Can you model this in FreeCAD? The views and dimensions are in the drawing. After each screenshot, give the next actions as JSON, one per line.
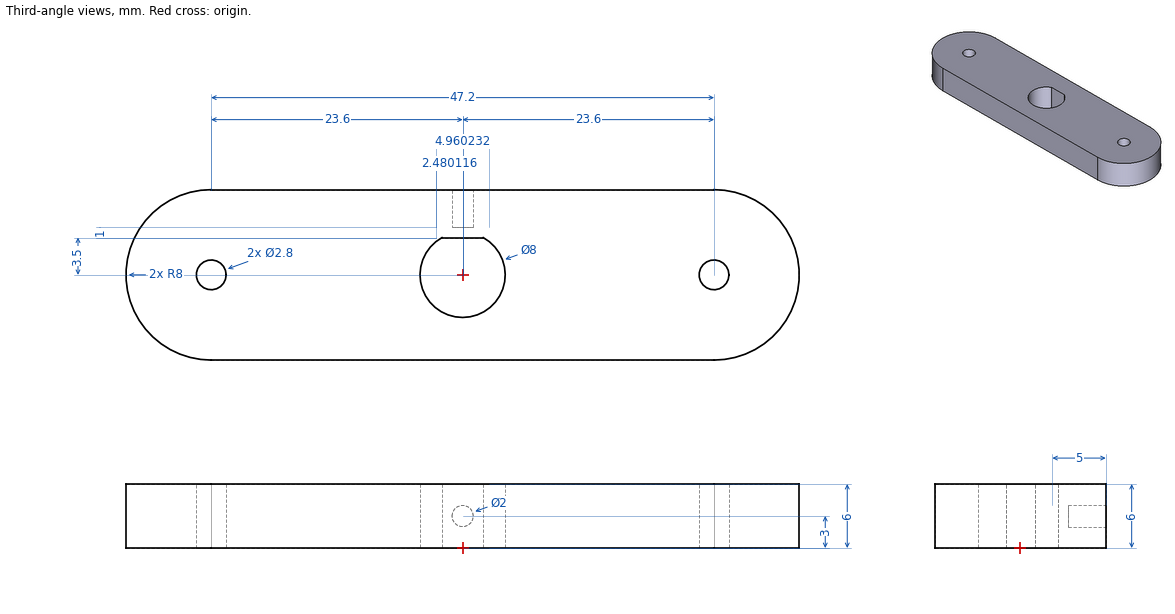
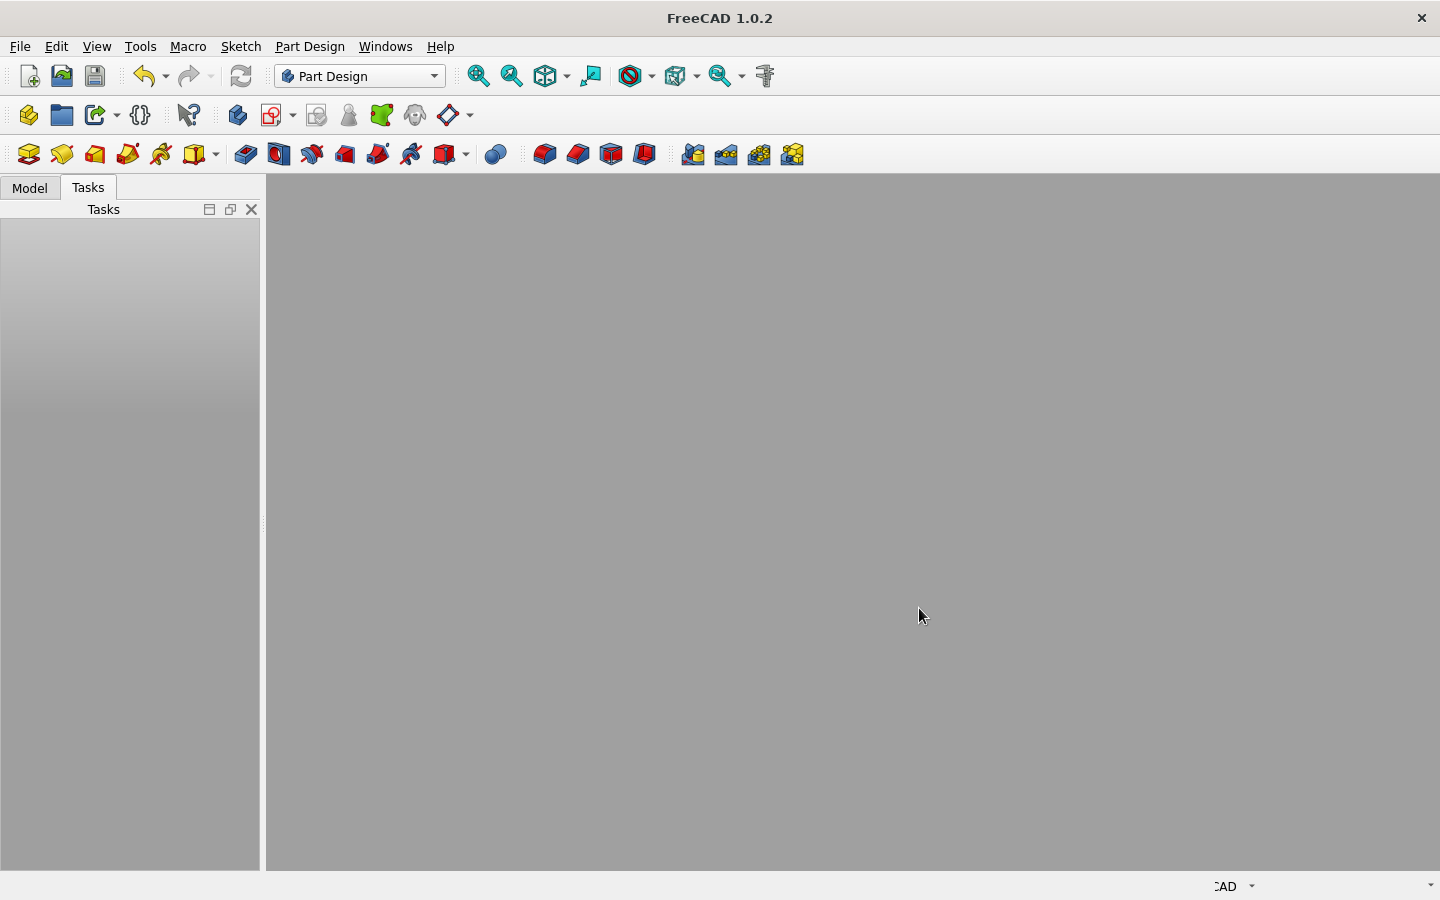
{"action": "left_click", "coordinate": [29, 76]}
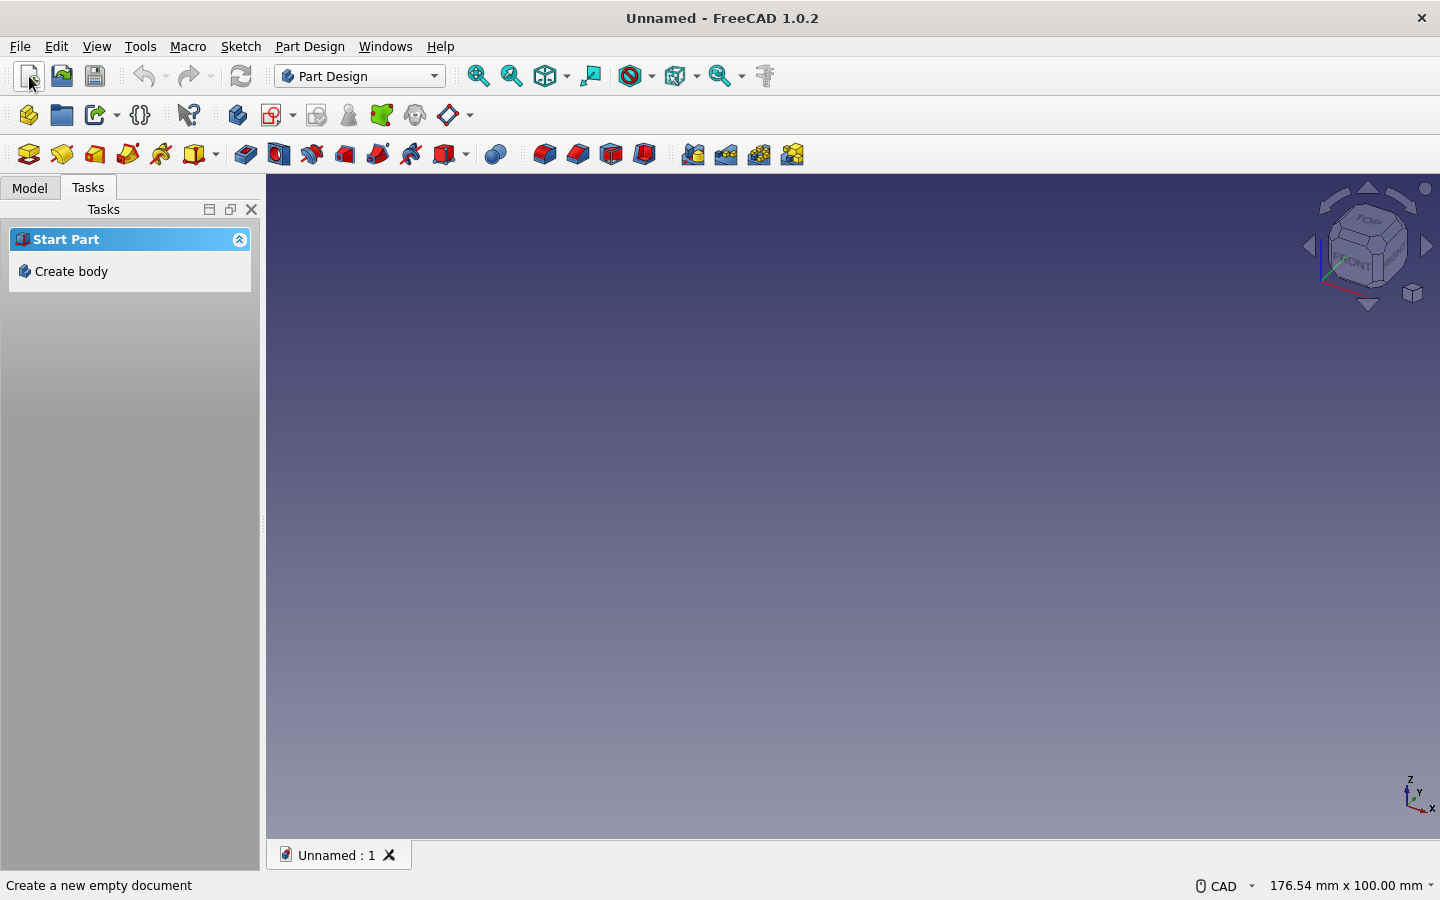
{"action": "left_click", "coordinate": [270, 116]}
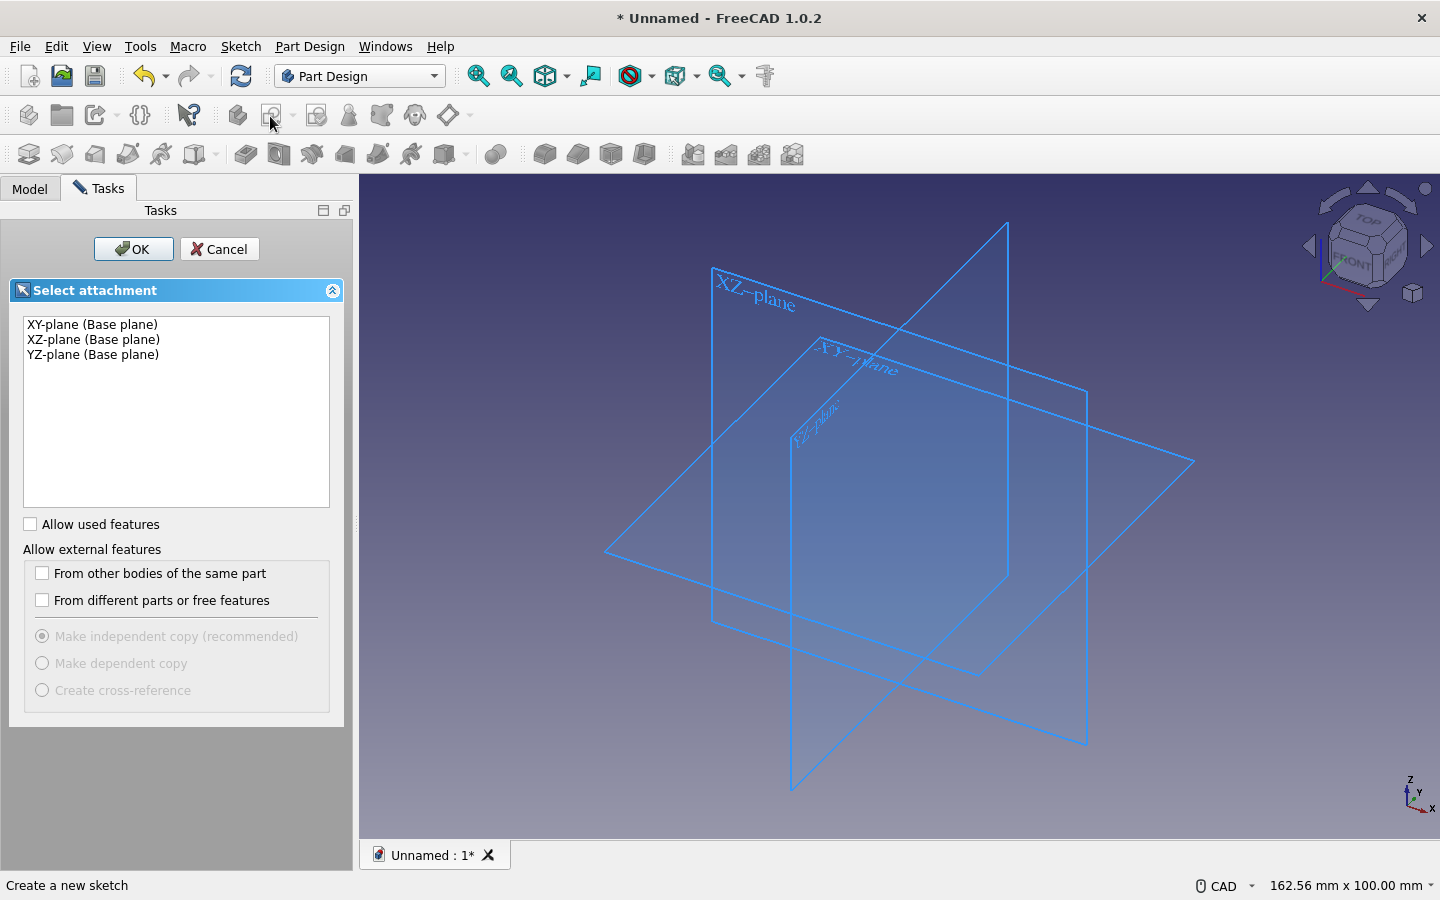
{"action": "left_click", "coordinate": [84, 324]}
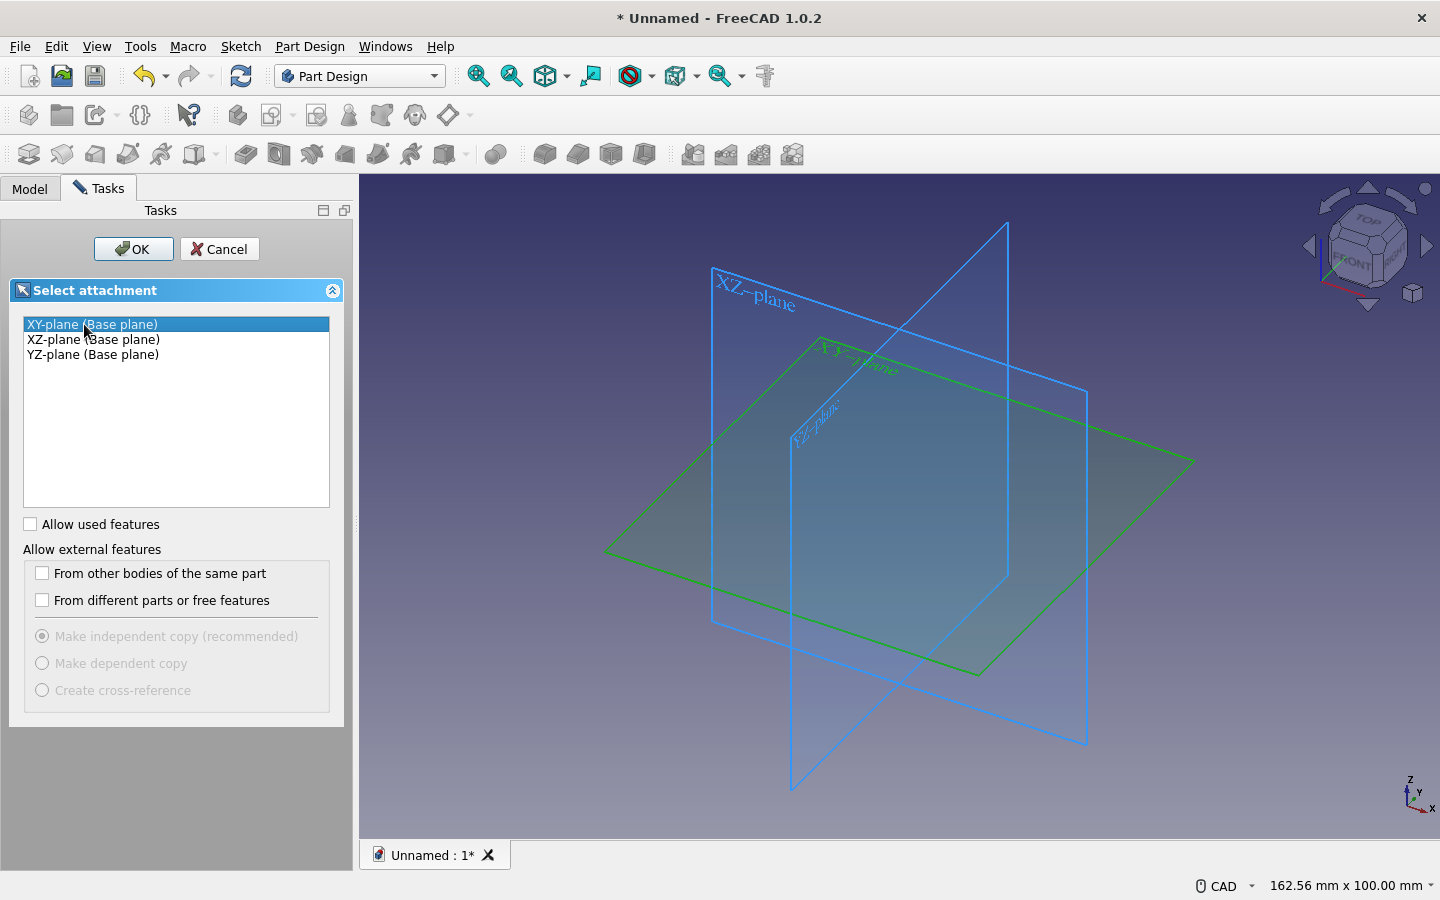
{"action": "left_click", "coordinate": [134, 249]}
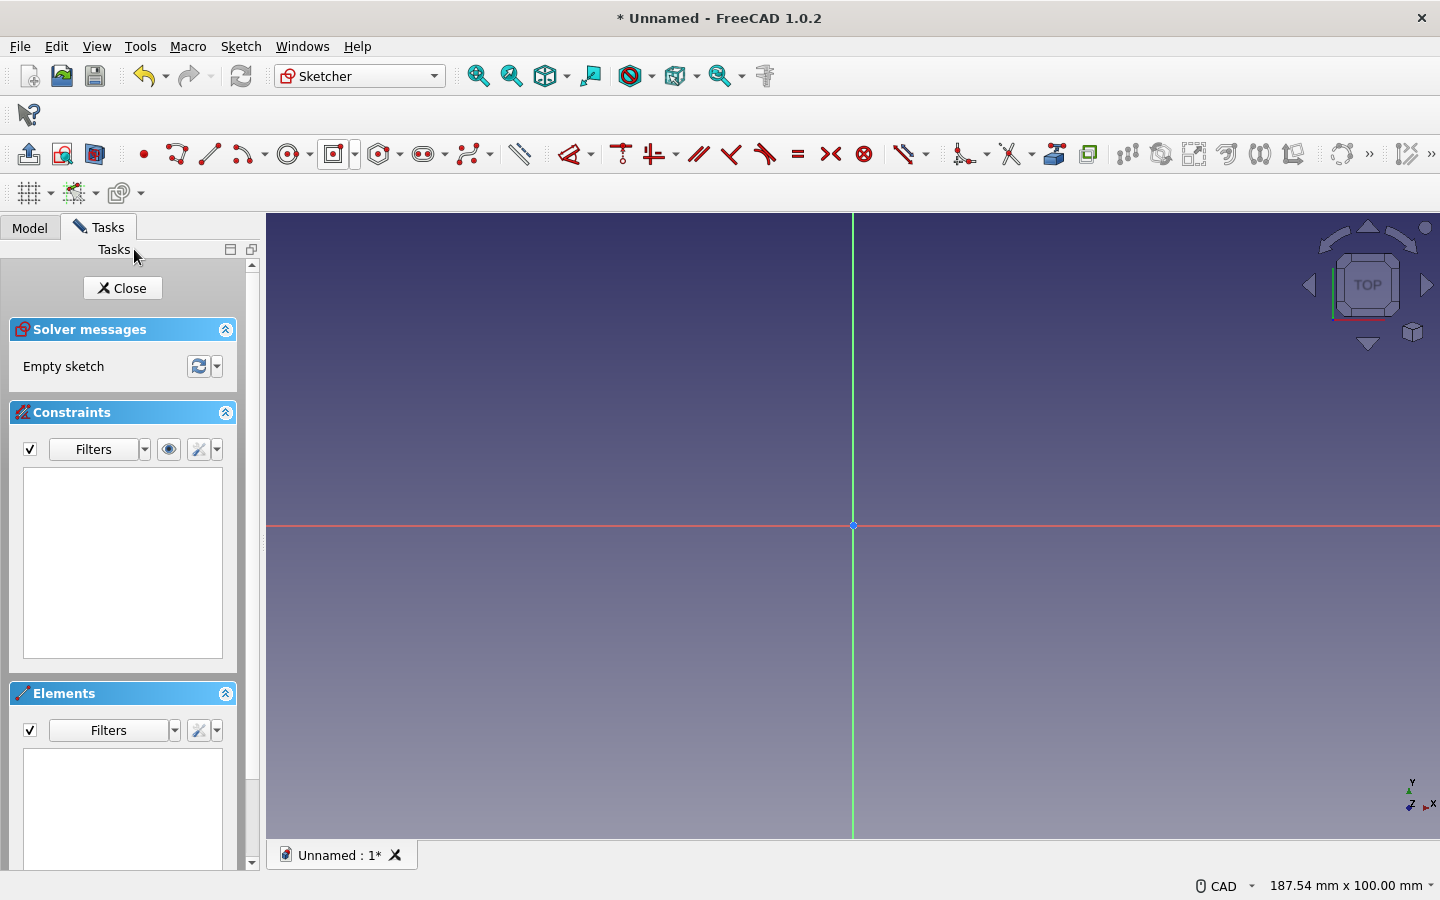
{"action": "scroll", "coordinate": [936, 526], "scroll_direction": "up", "scroll_amount": 3}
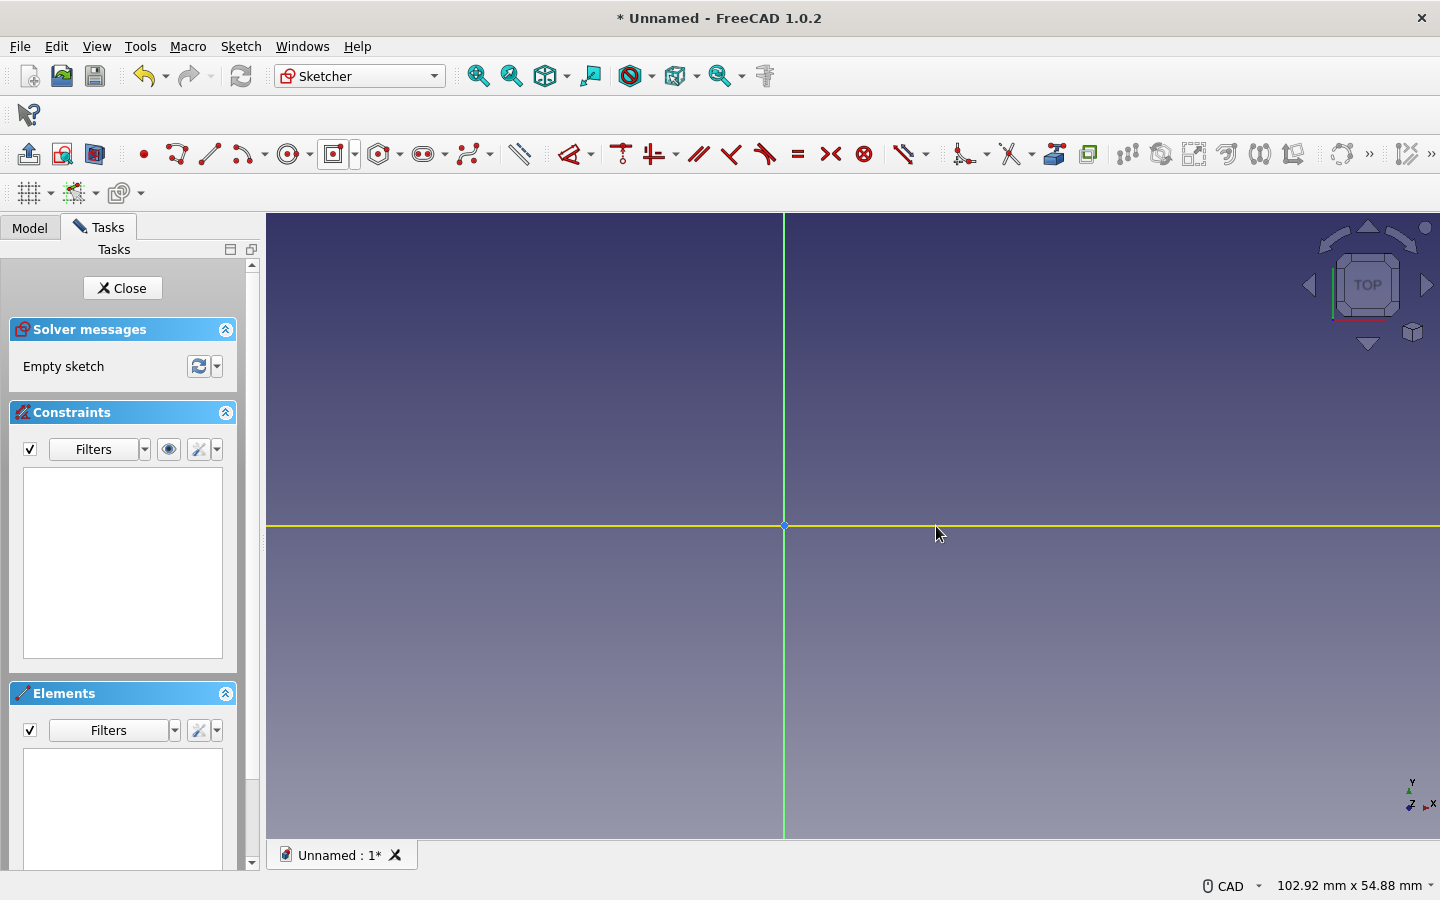
{"action": "left_click", "coordinate": [422, 154]}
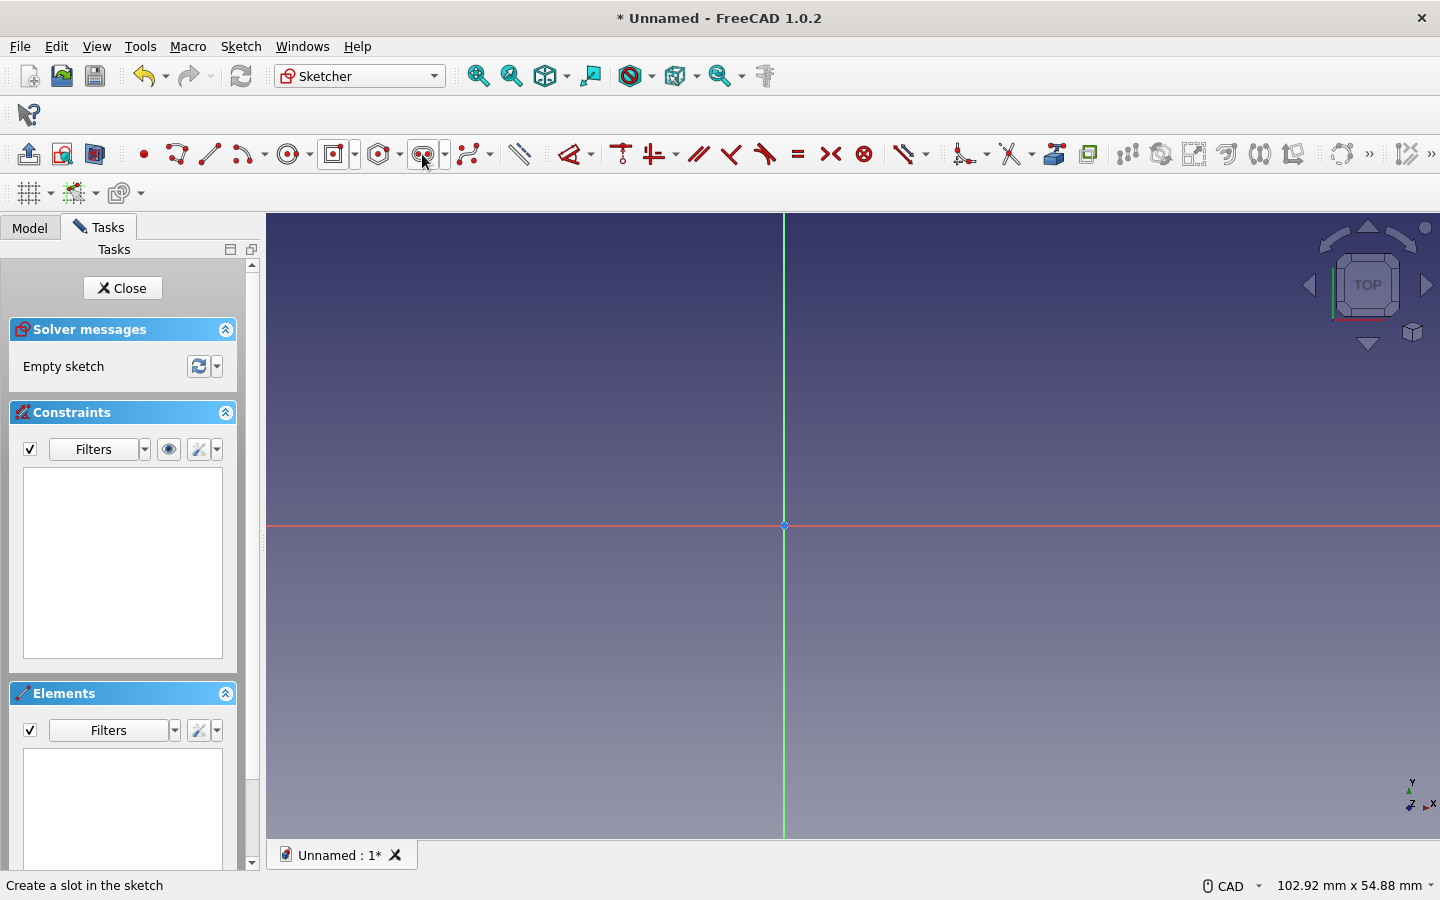
{"action": "left_click", "coordinate": [515, 526]}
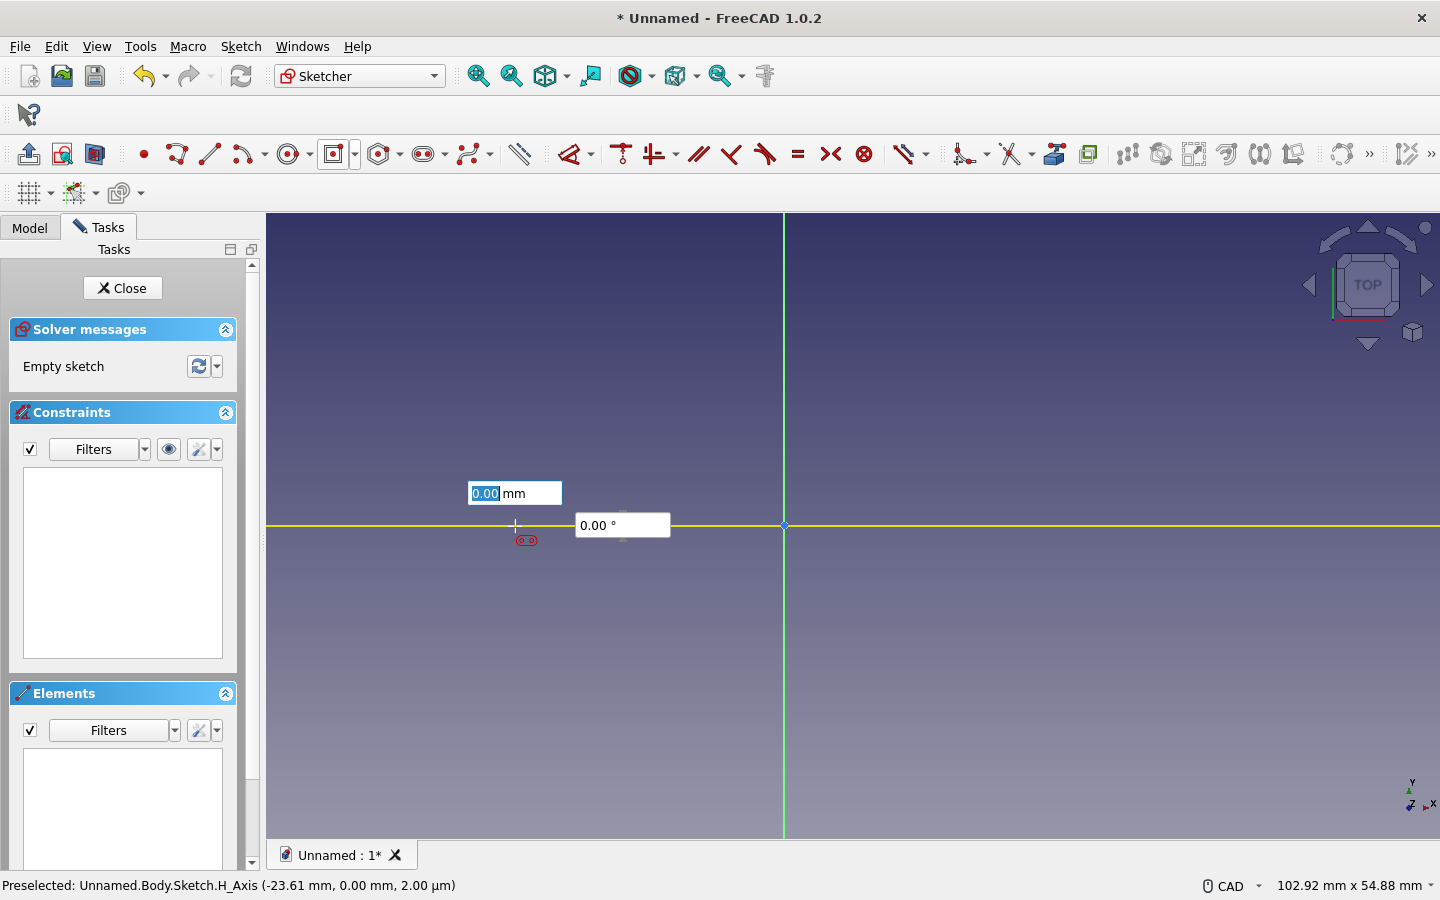
{"action": "left_click", "coordinate": [1053, 517]}